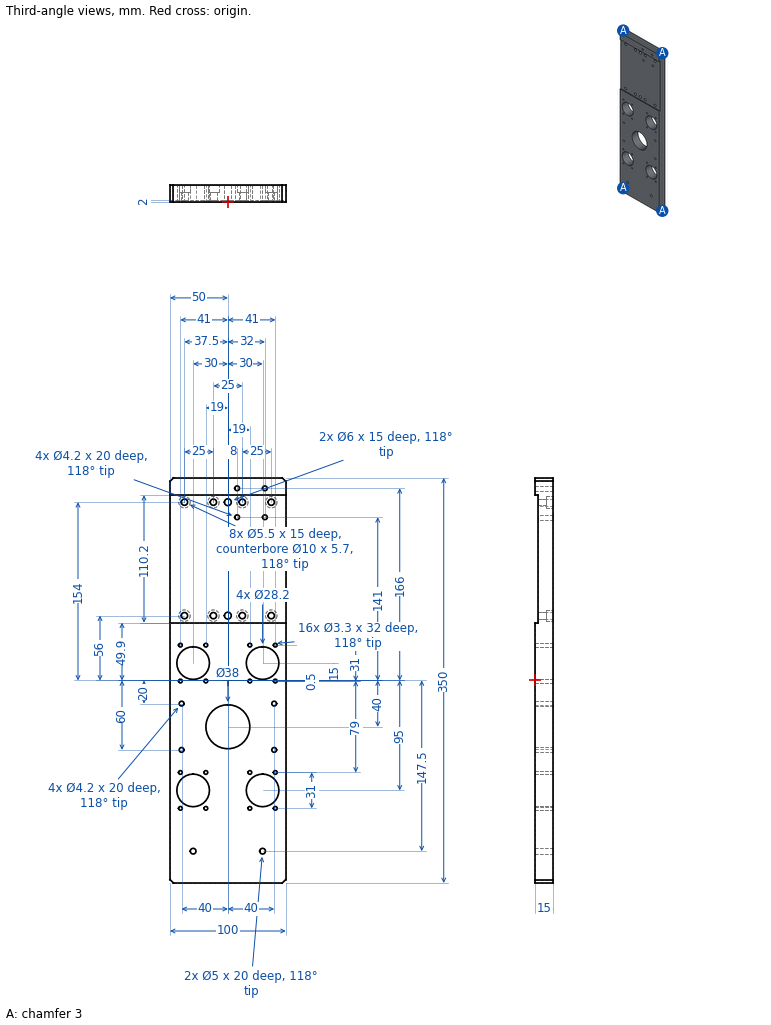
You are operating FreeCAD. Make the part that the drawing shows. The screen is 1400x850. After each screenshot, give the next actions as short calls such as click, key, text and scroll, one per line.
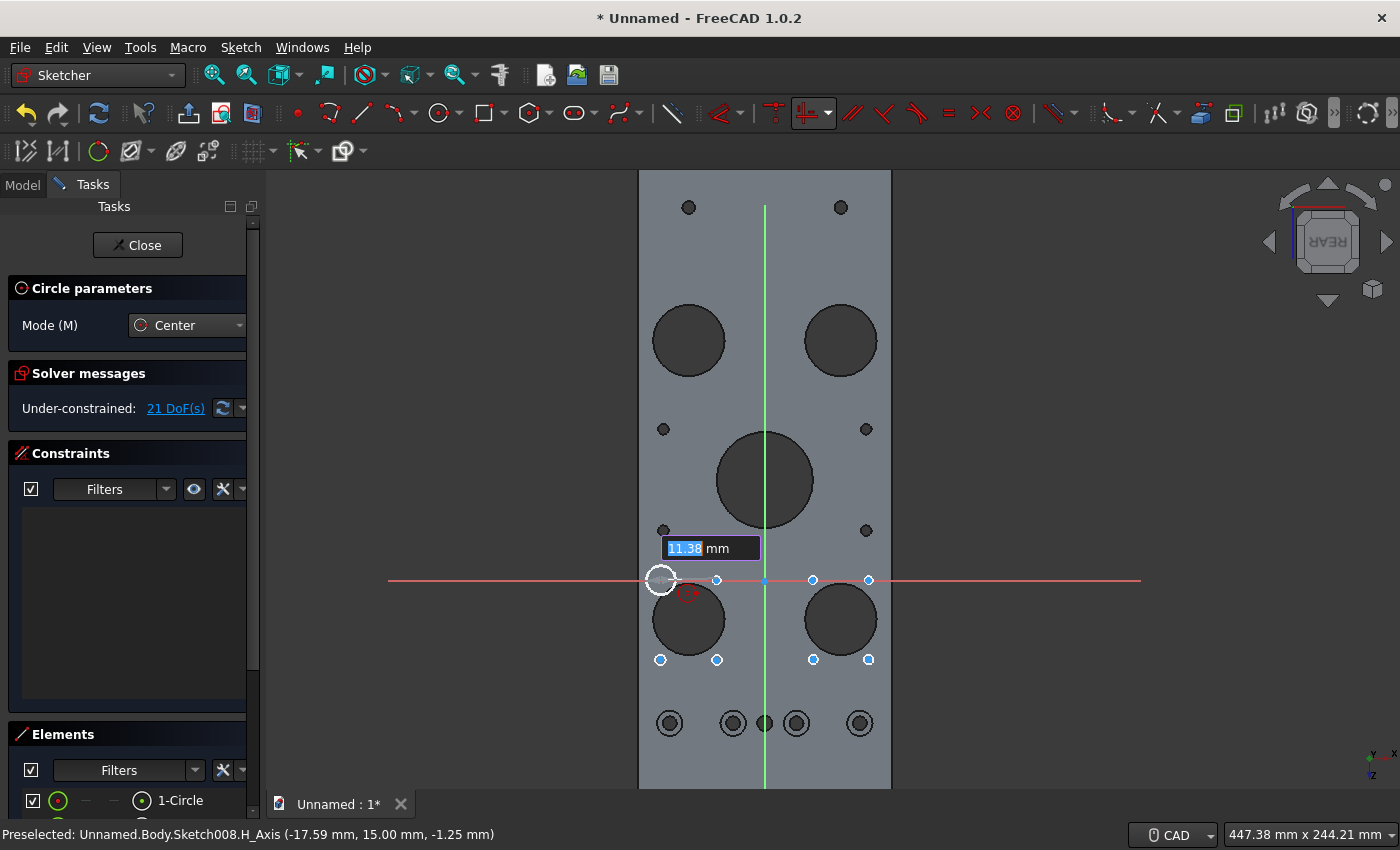
scroll(664, 577, up, 7)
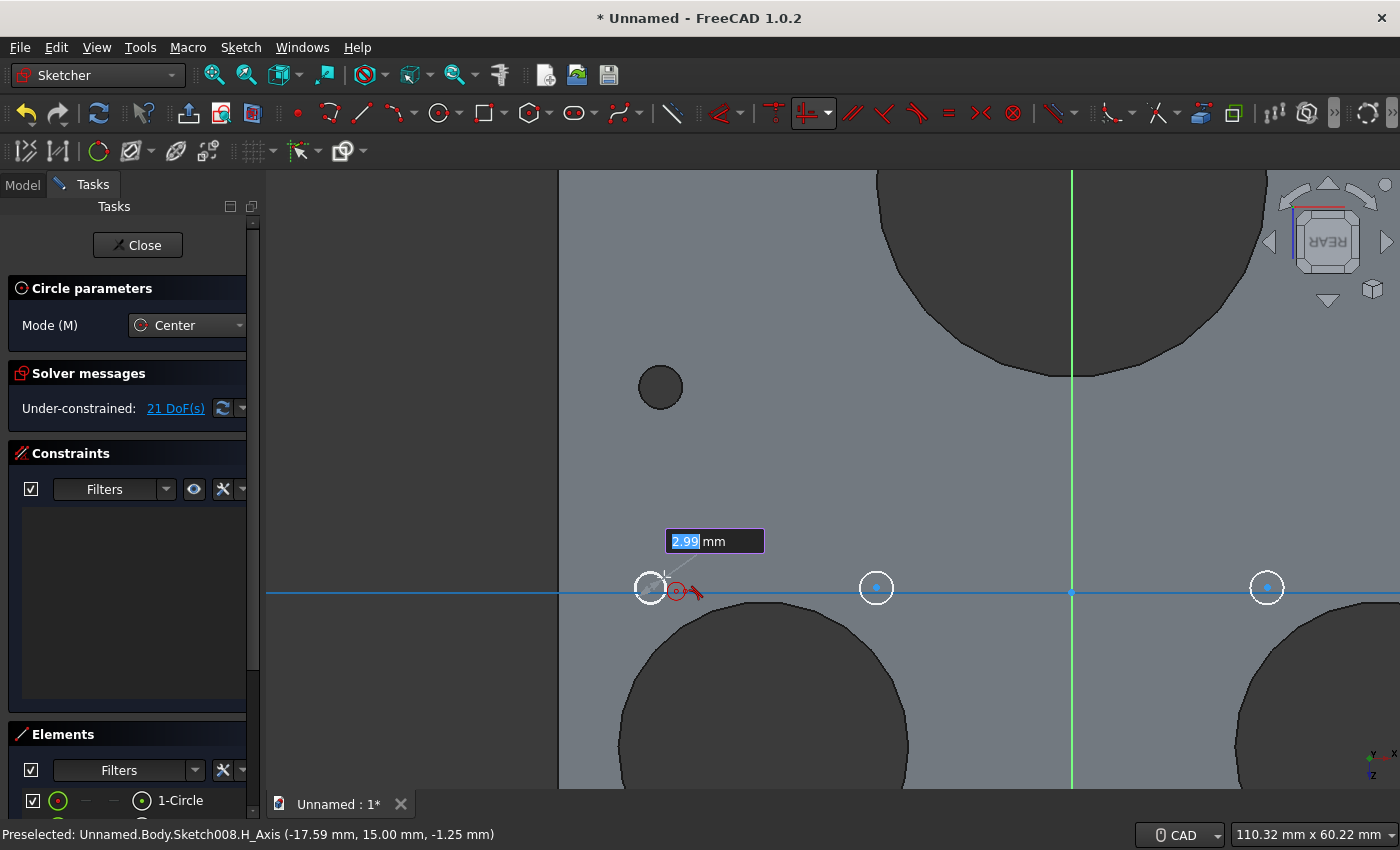
click(662, 576)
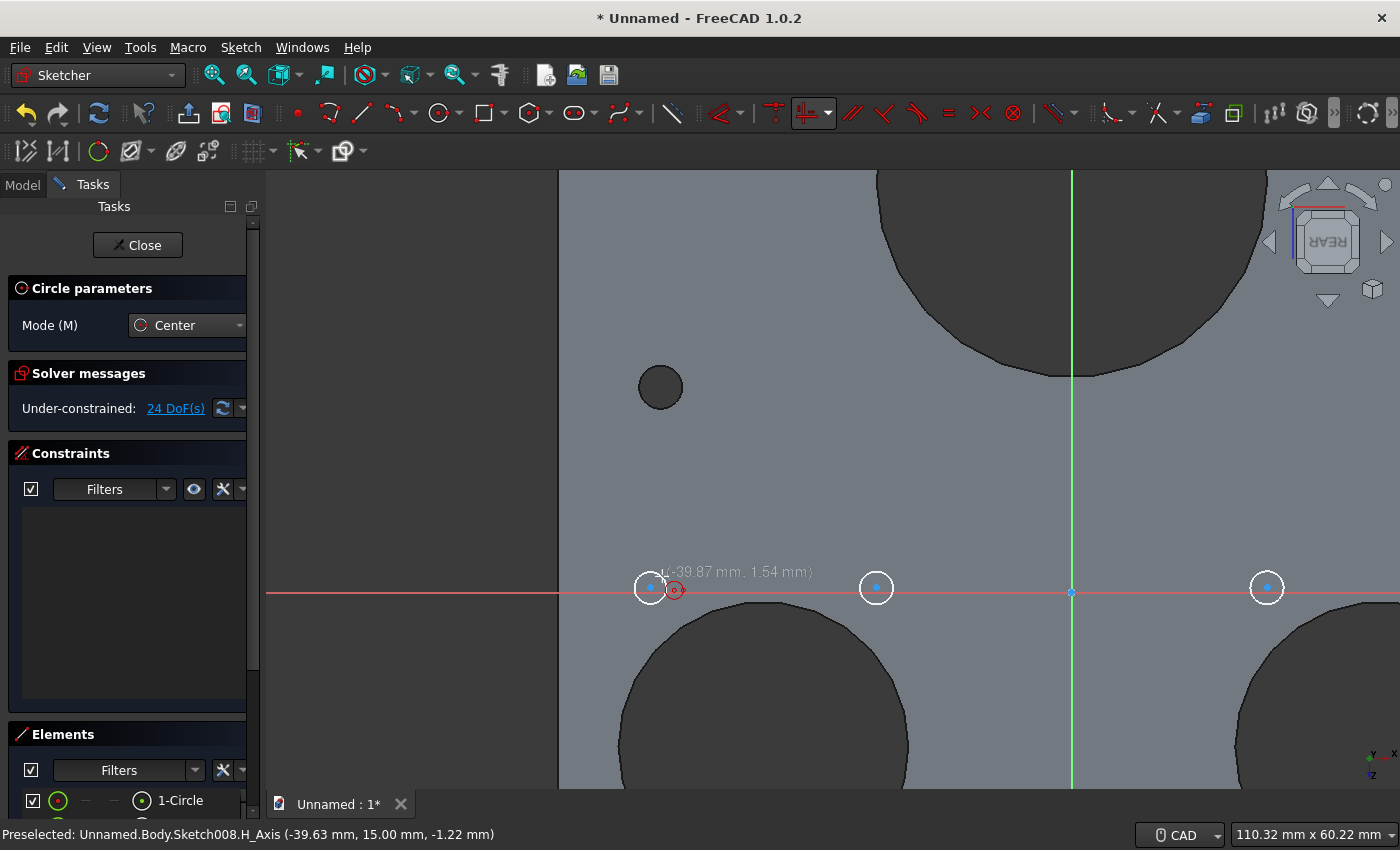
scroll(664, 577, down, 7)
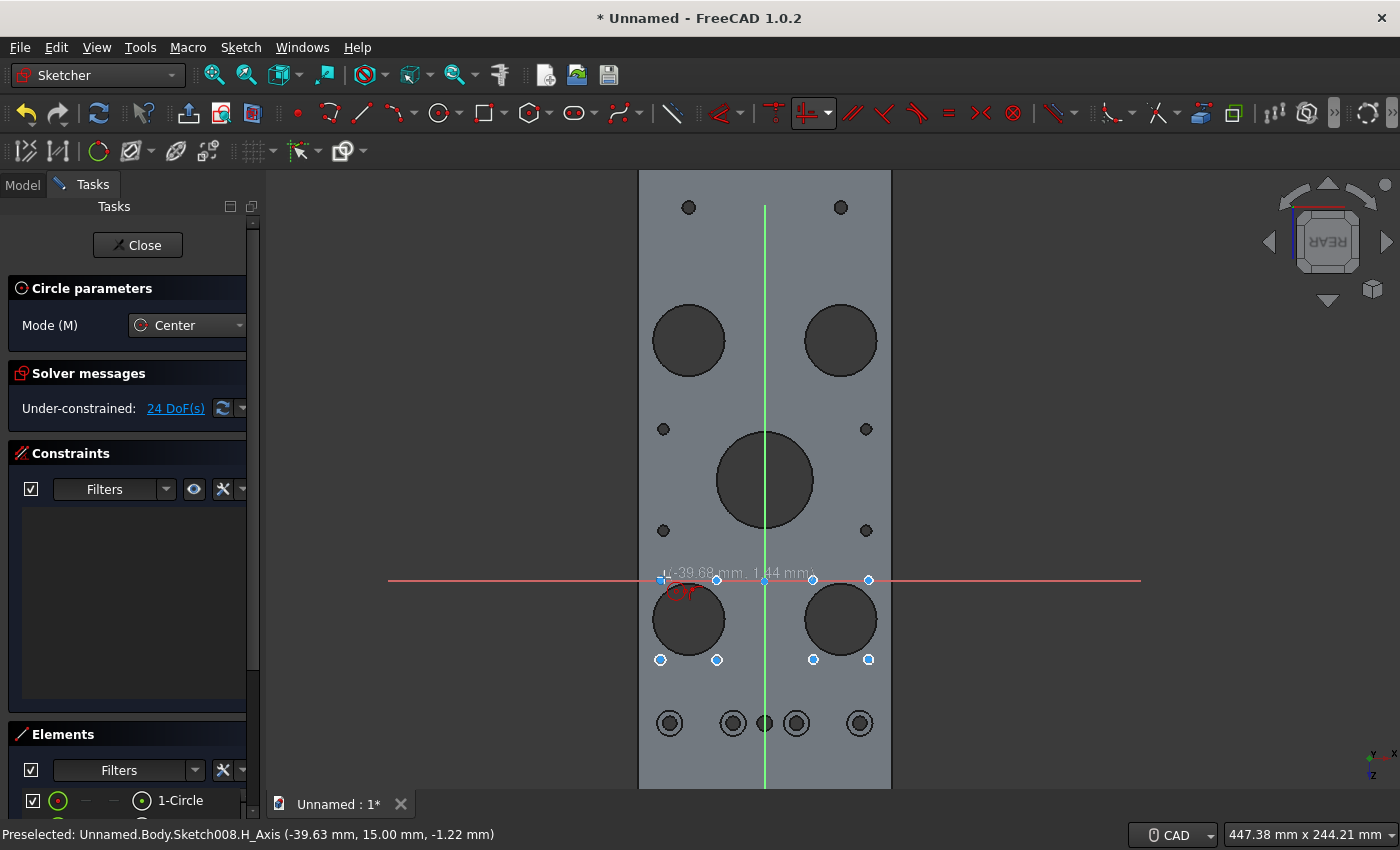
scroll(869, 380, up, 9)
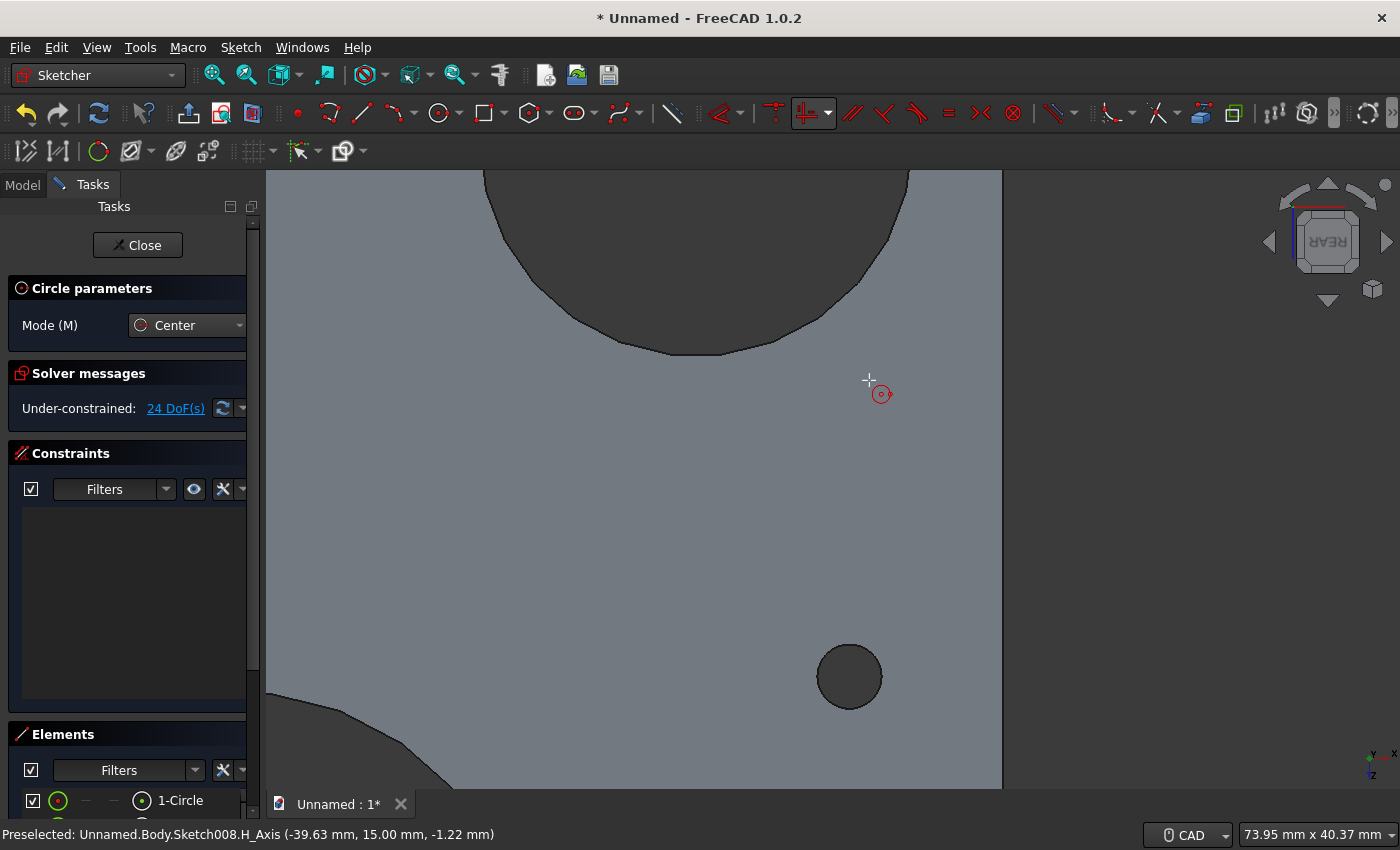
scroll(869, 380, down, 9)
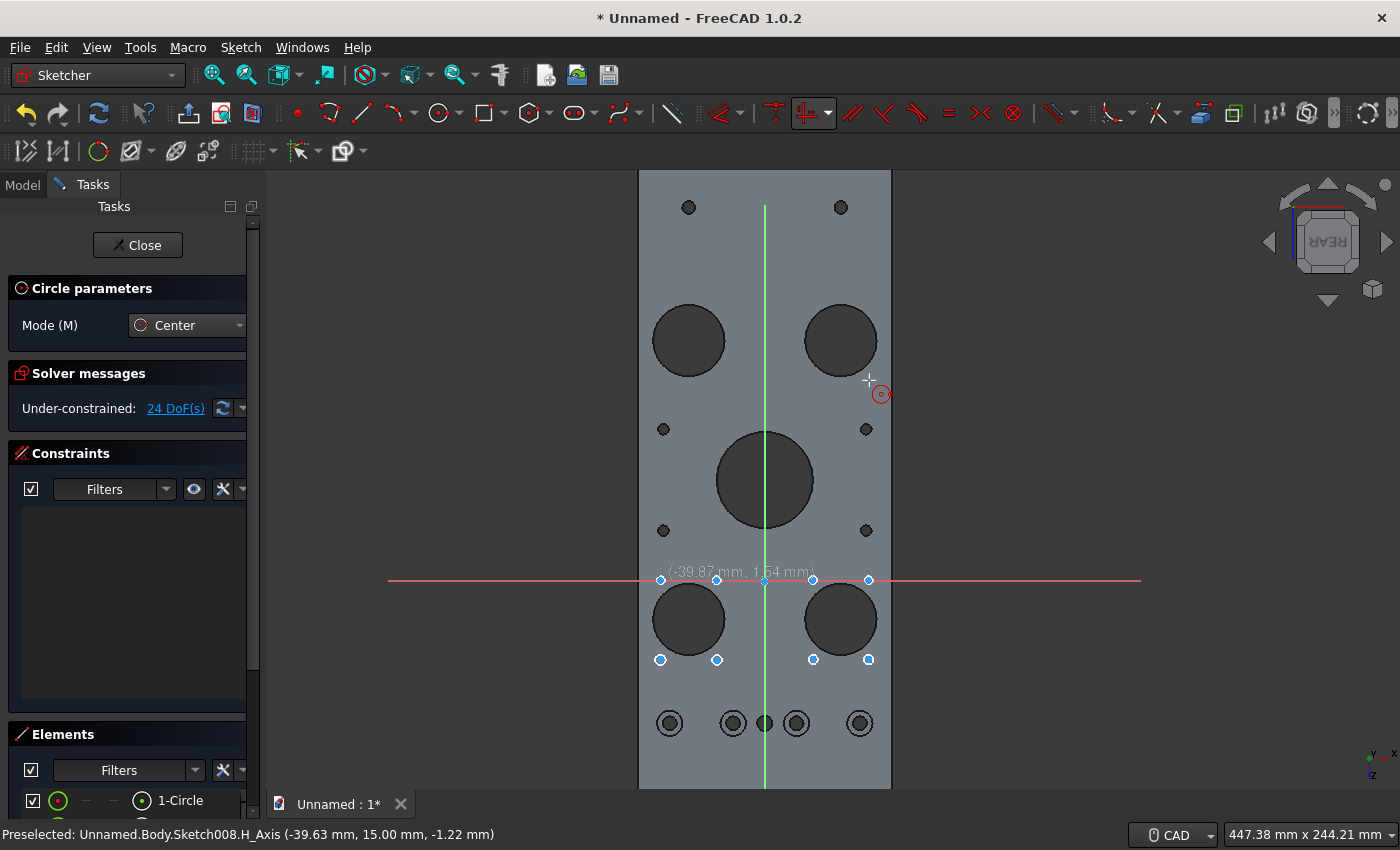
click(869, 380)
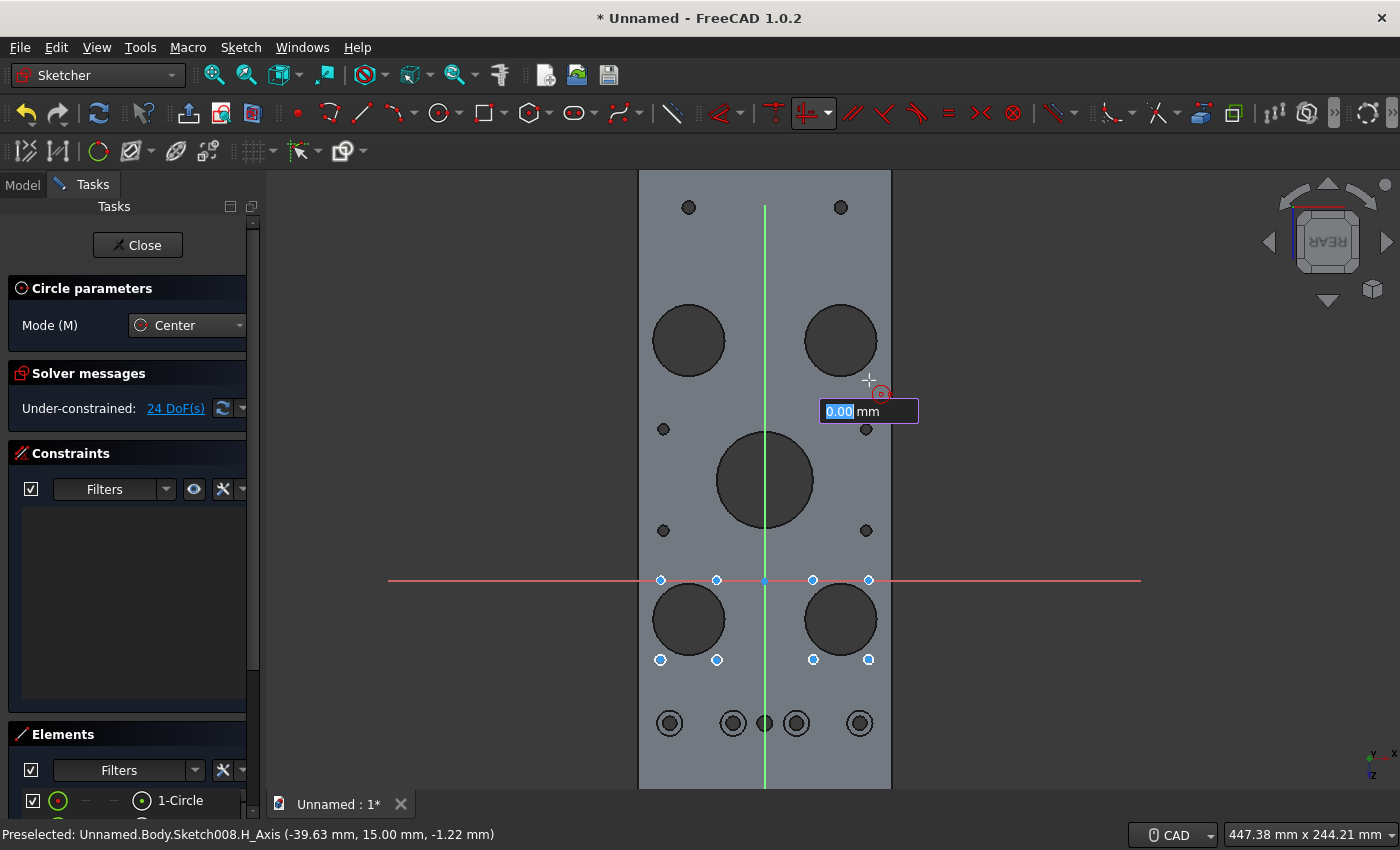
scroll(872, 377, up, 7)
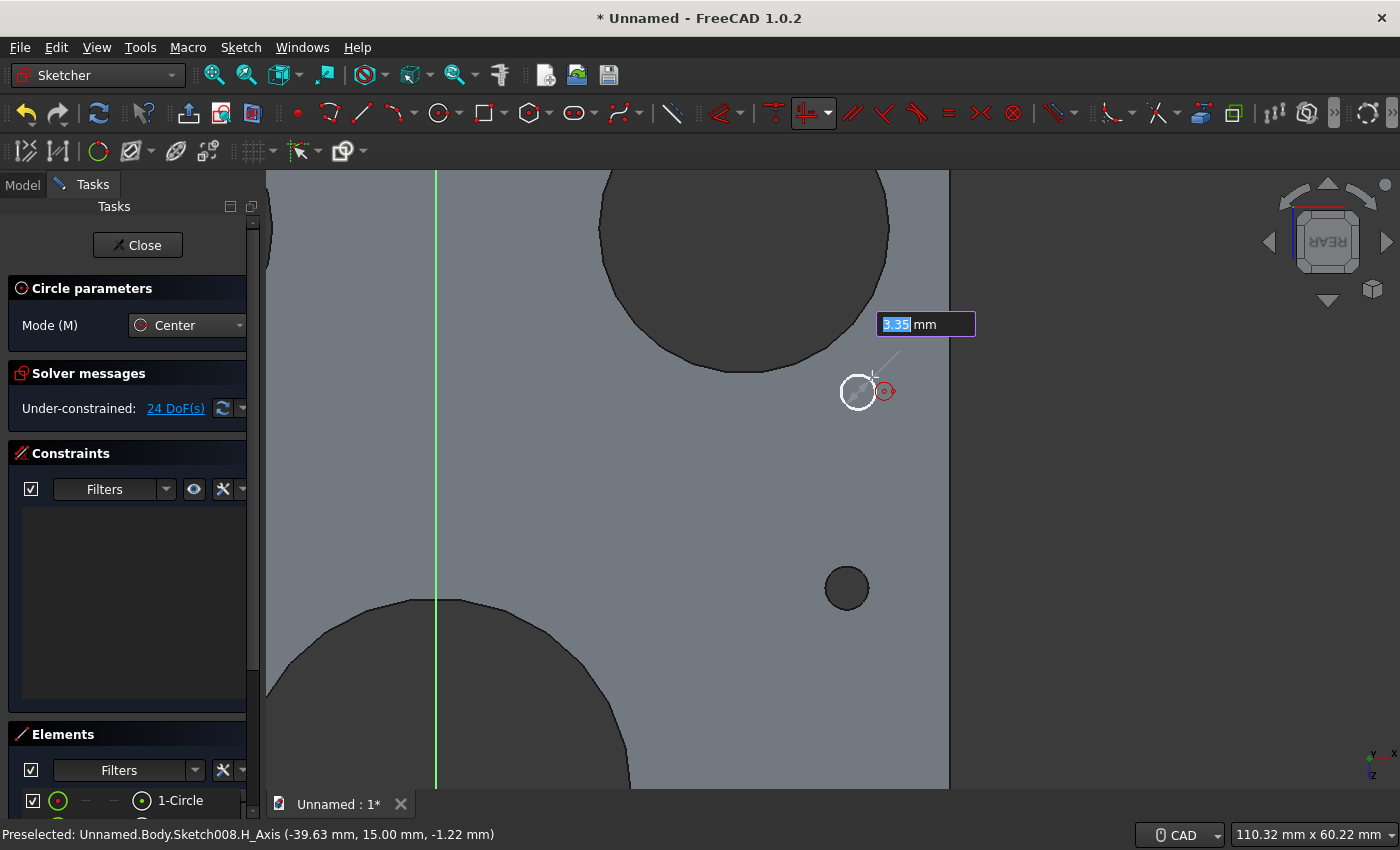
click(869, 376)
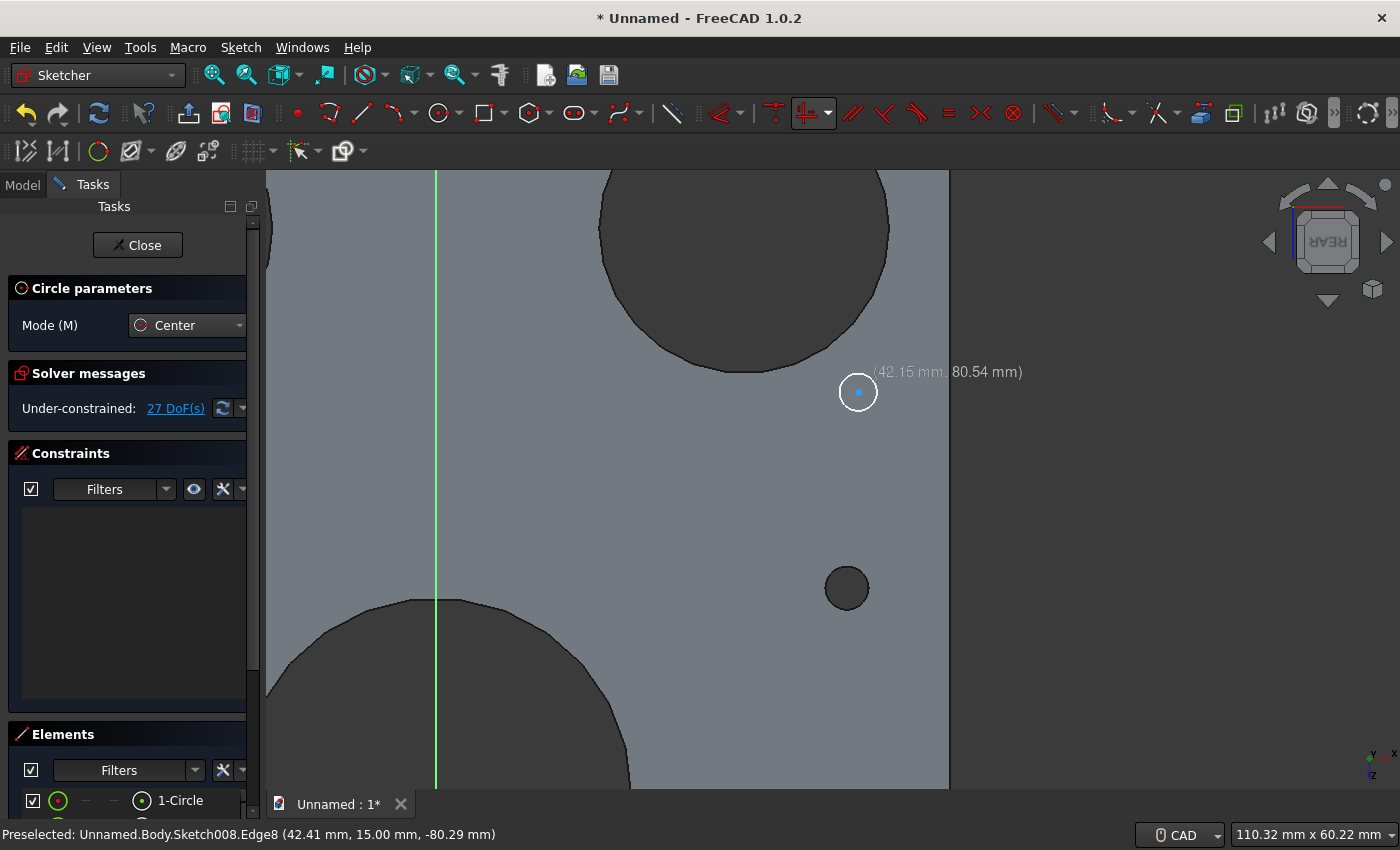
scroll(631, 388, up, 2)